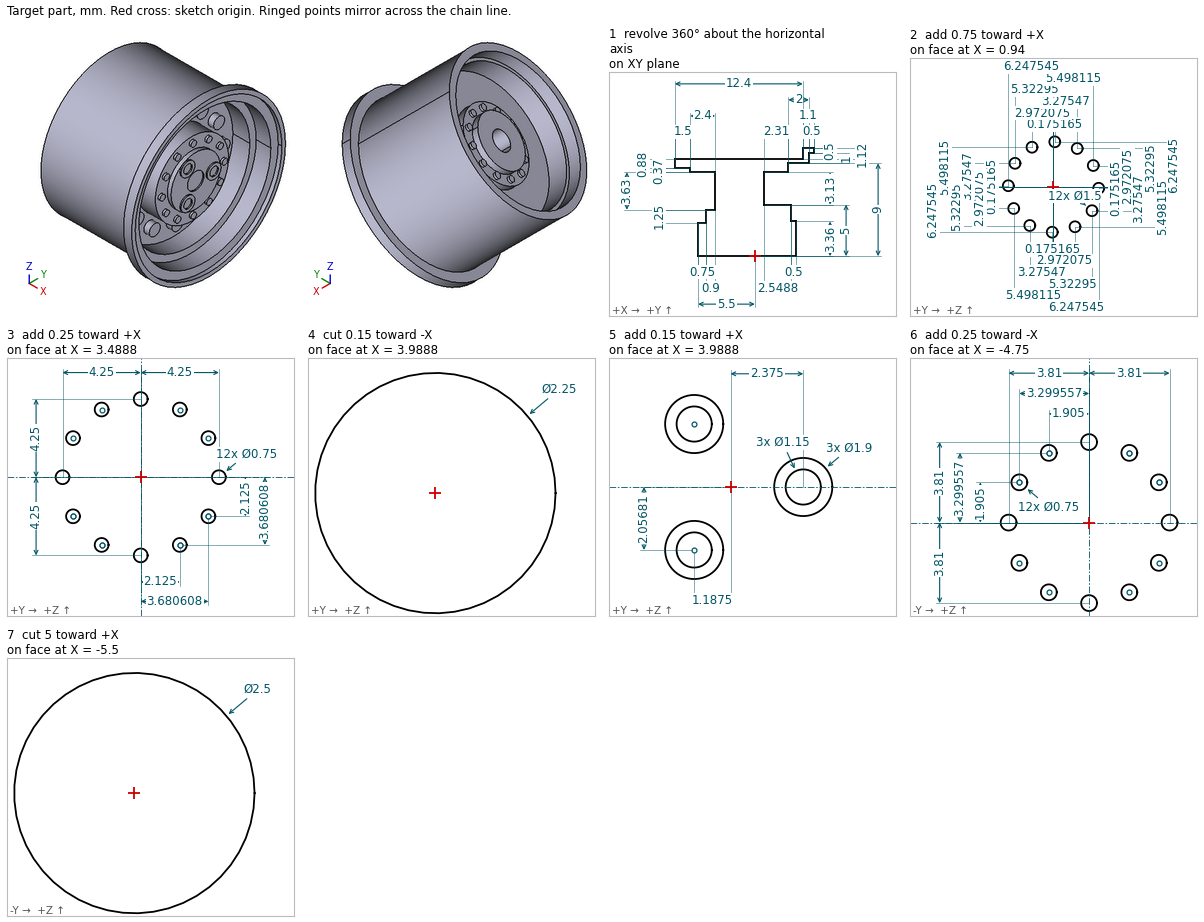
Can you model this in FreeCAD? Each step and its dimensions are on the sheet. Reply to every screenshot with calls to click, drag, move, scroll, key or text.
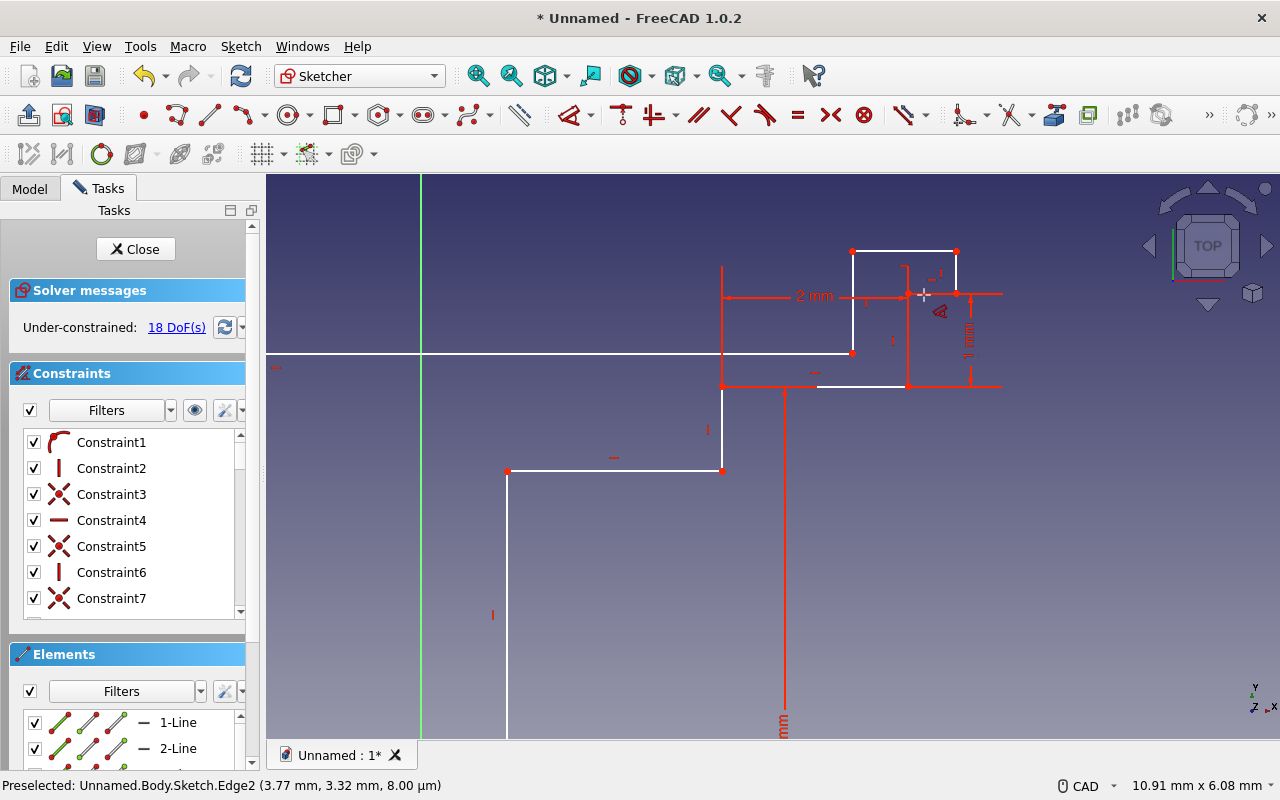
click(922, 294)
click(932, 236)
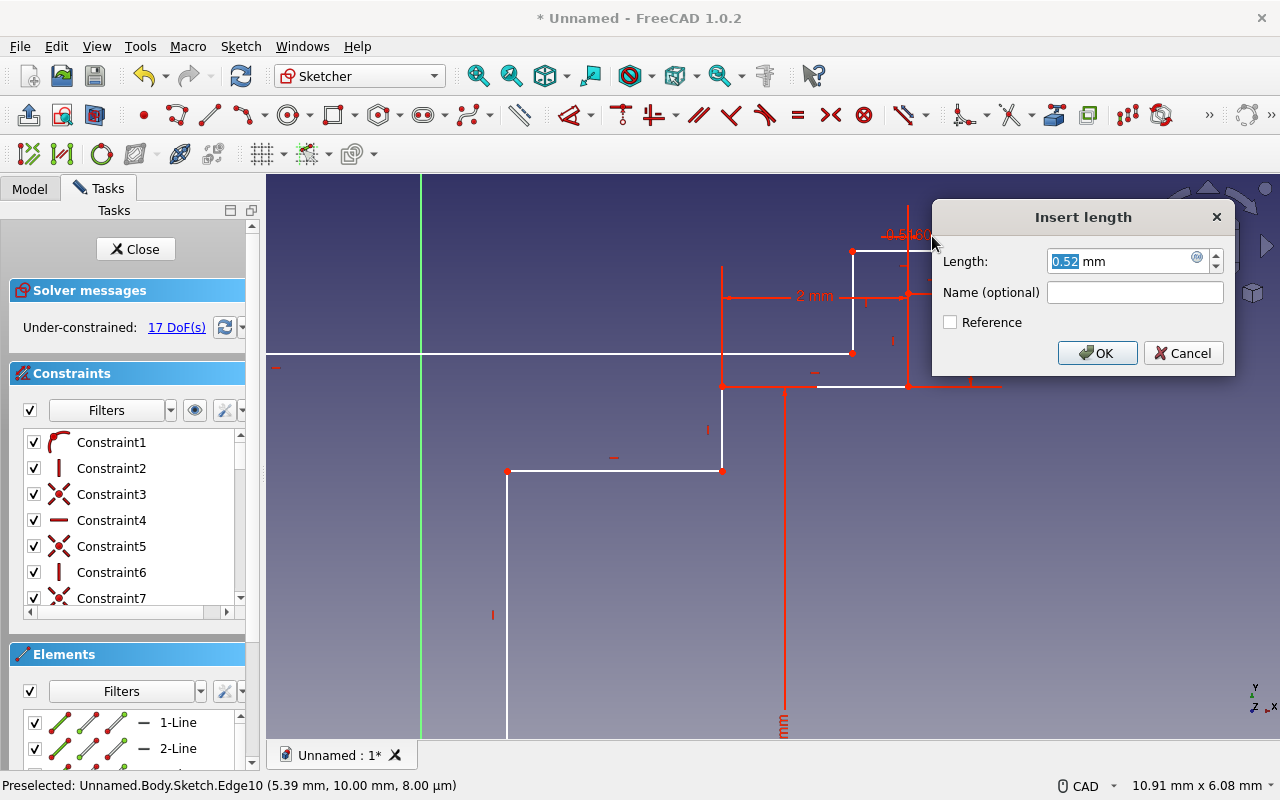
text(0.5)
key(Return)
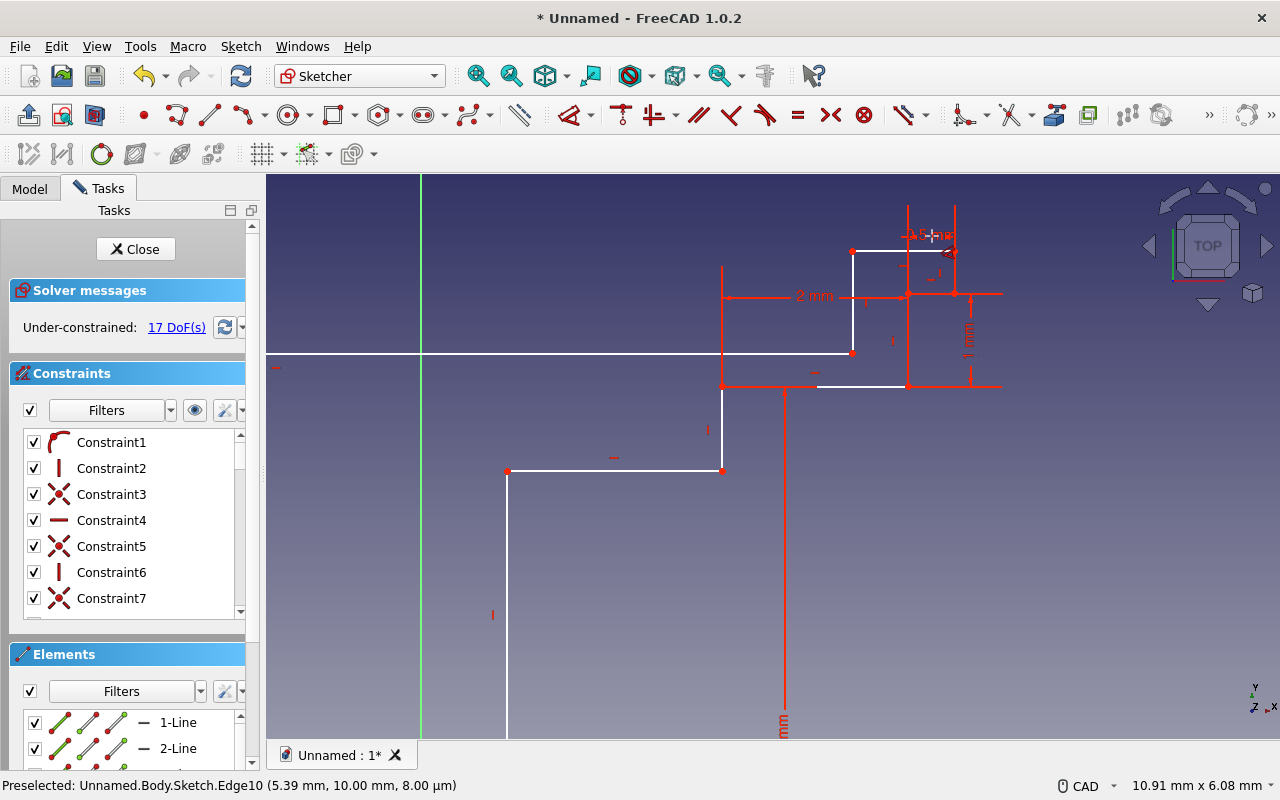
click(955, 281)
click(989, 273)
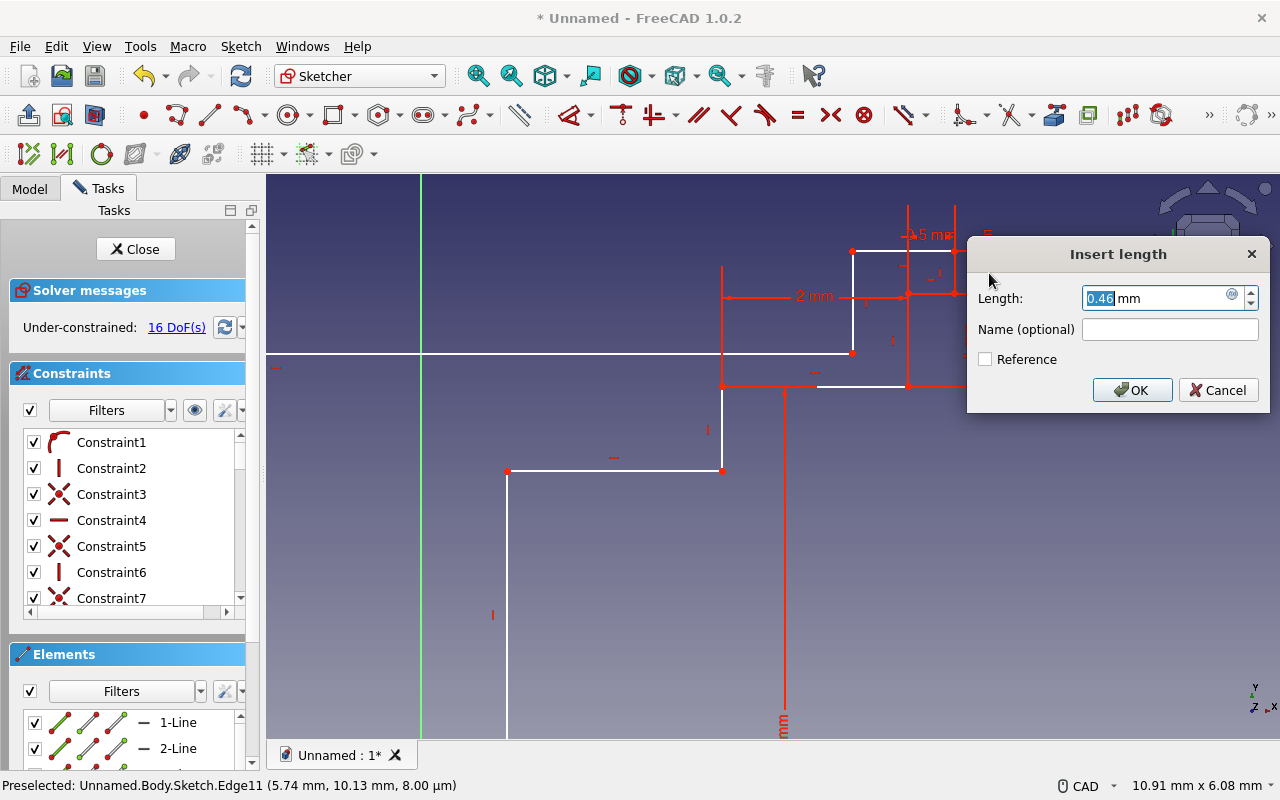
text(0.5)
key(Return)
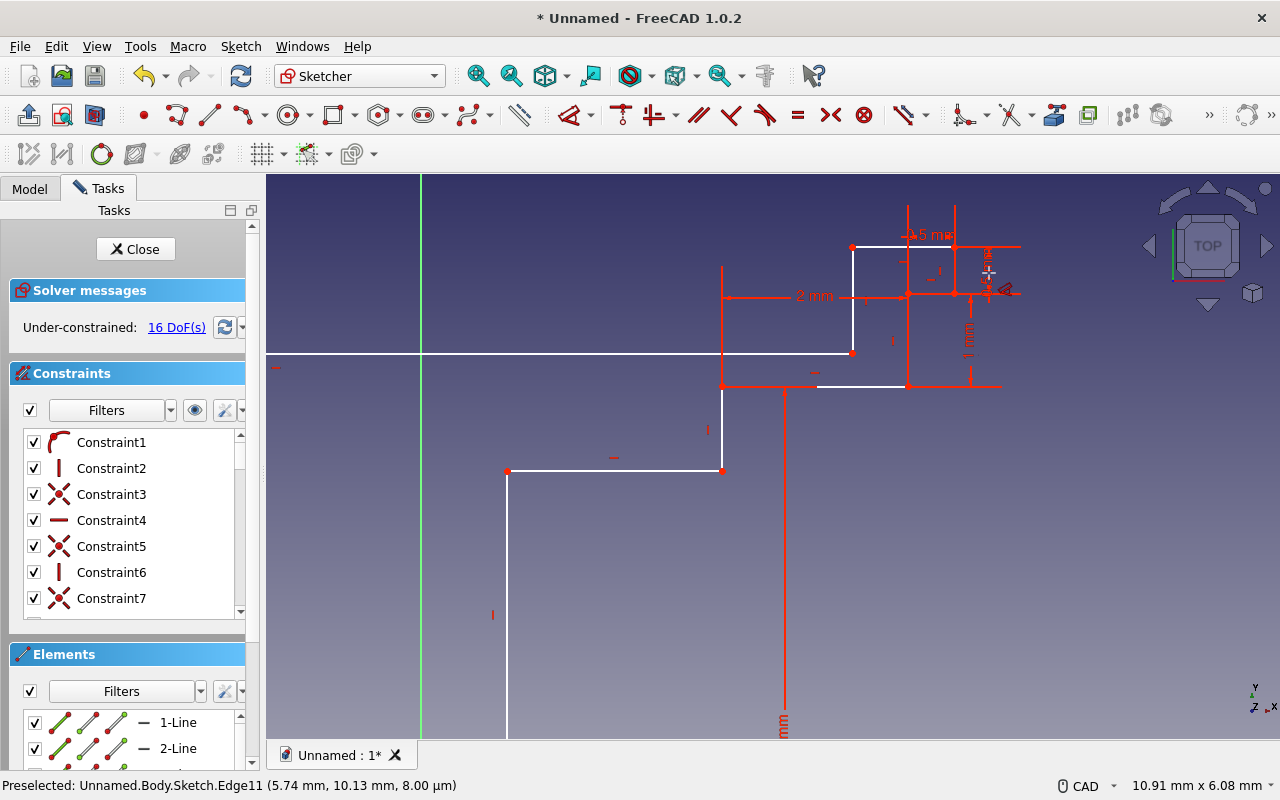
click(924, 247)
click(904, 213)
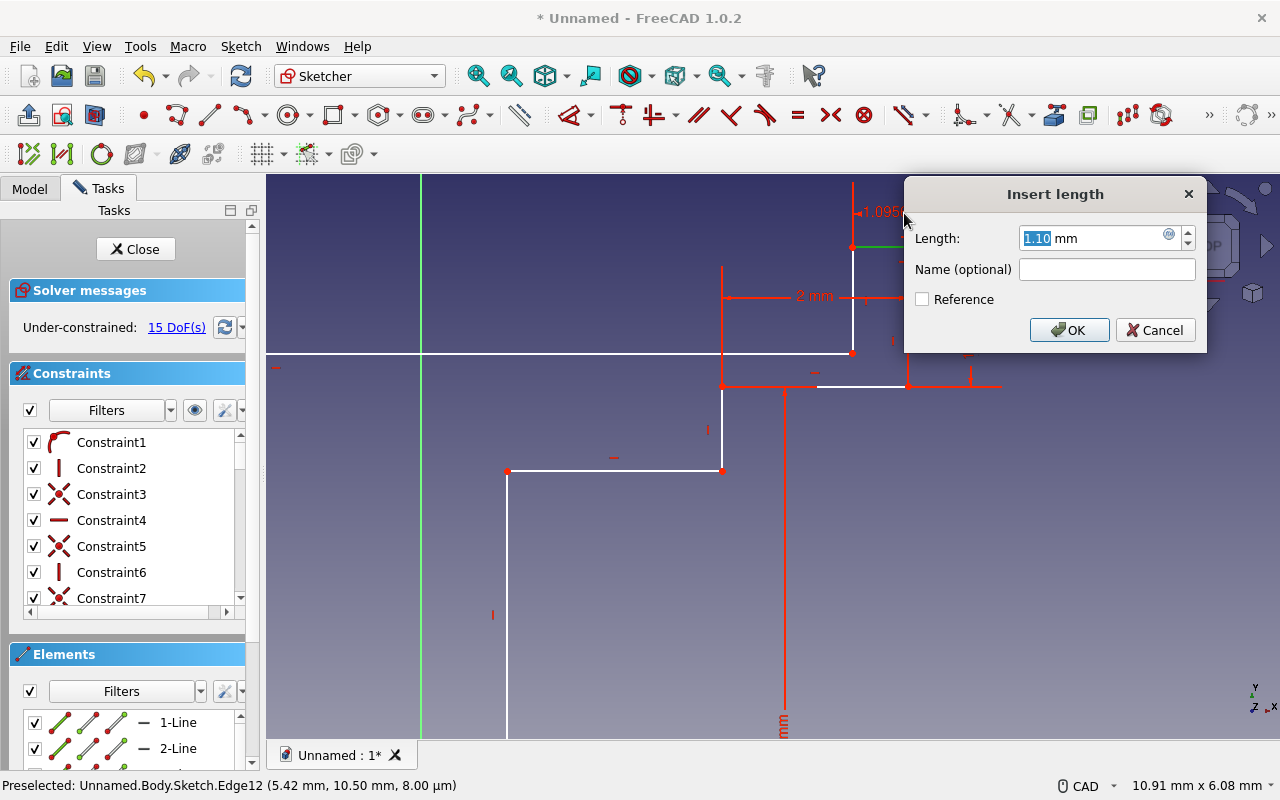
text(1.1)
key(Return)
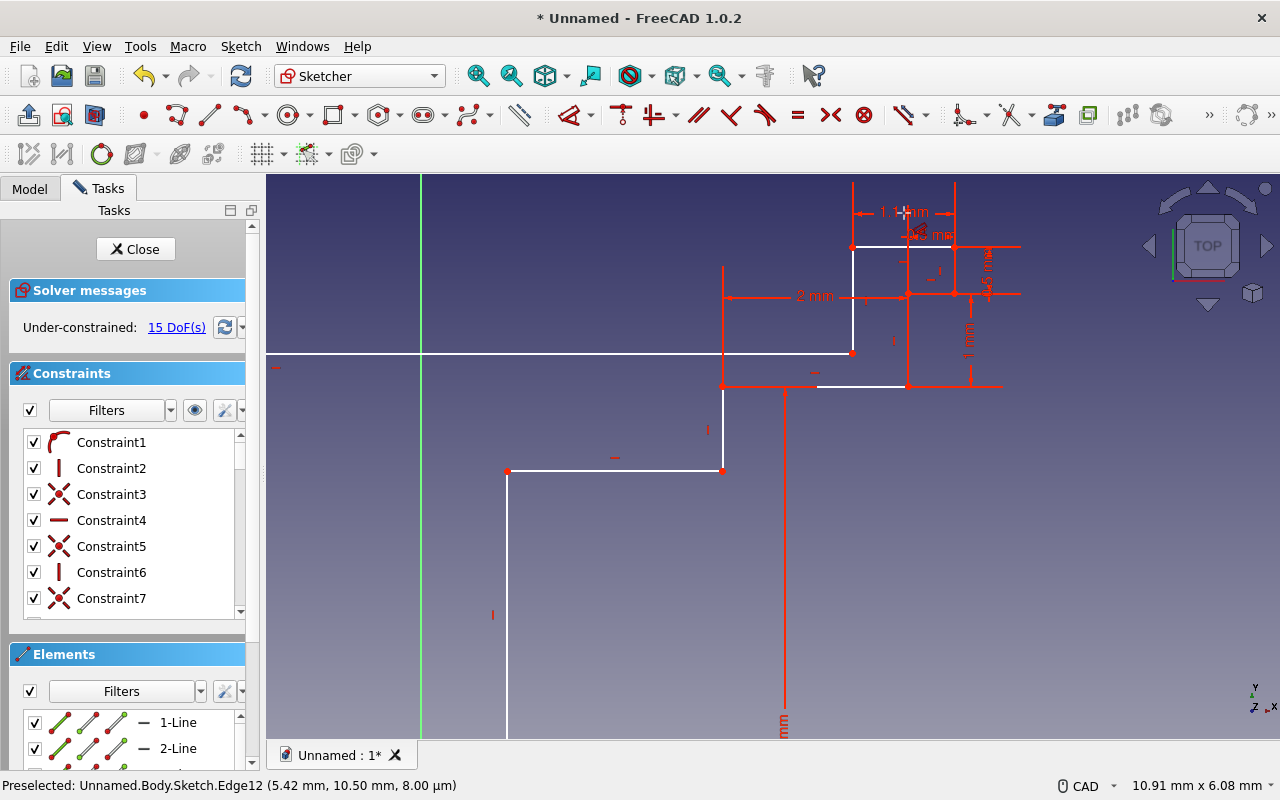
scroll(924, 294, down, 5)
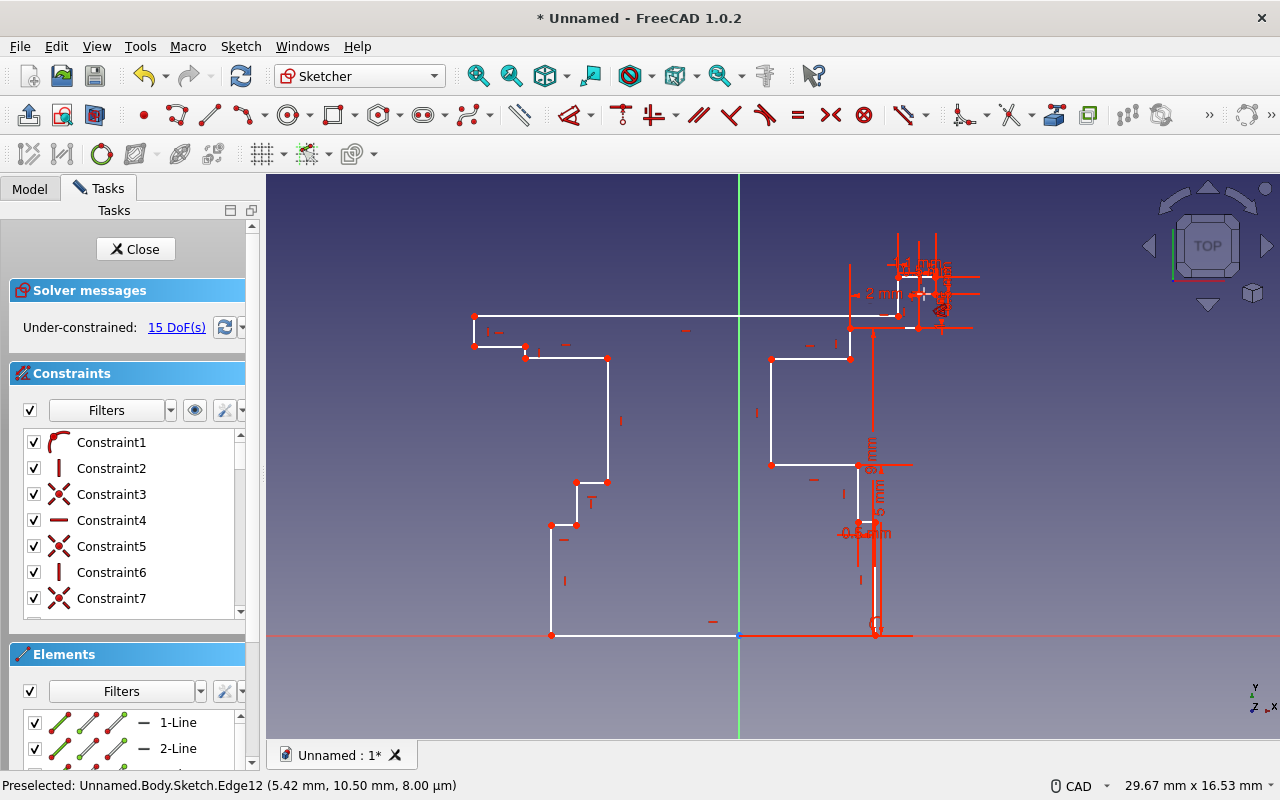
click(490, 347)
click(500, 381)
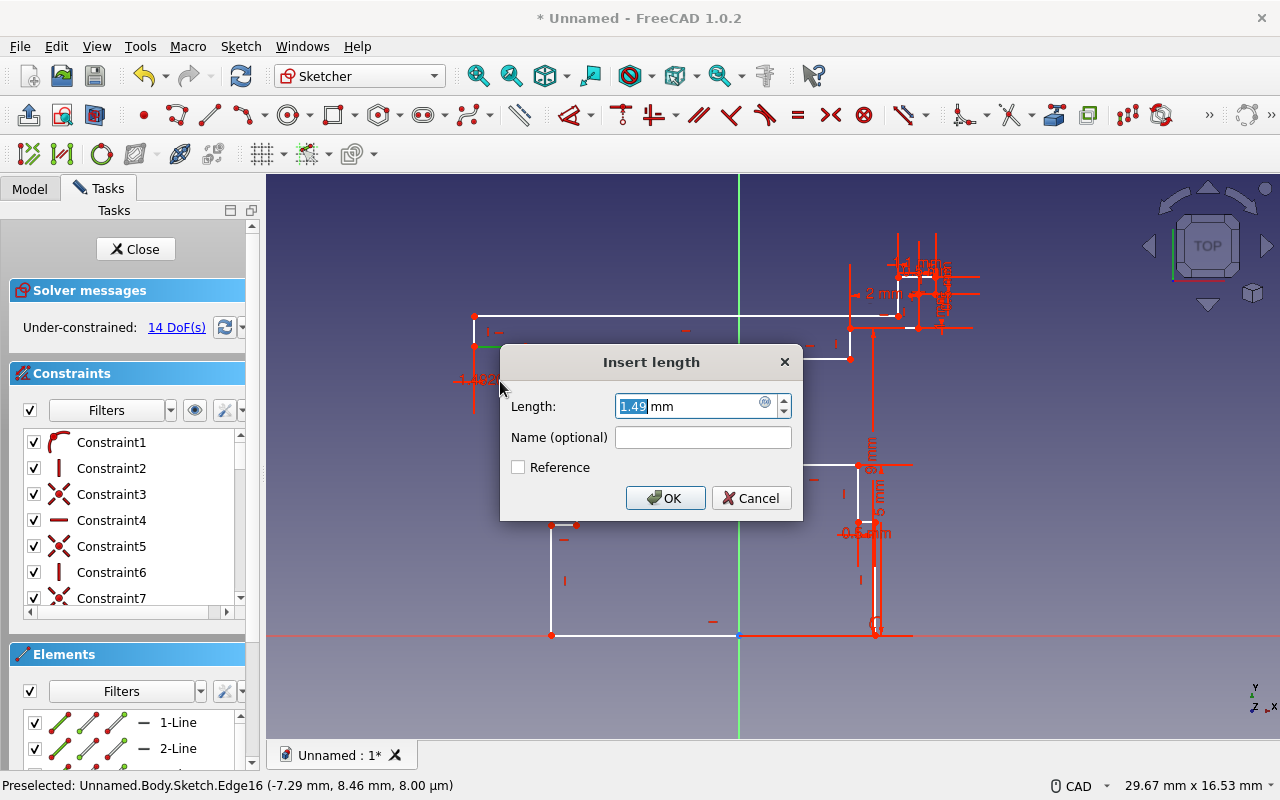
text(1.5)
key(Return)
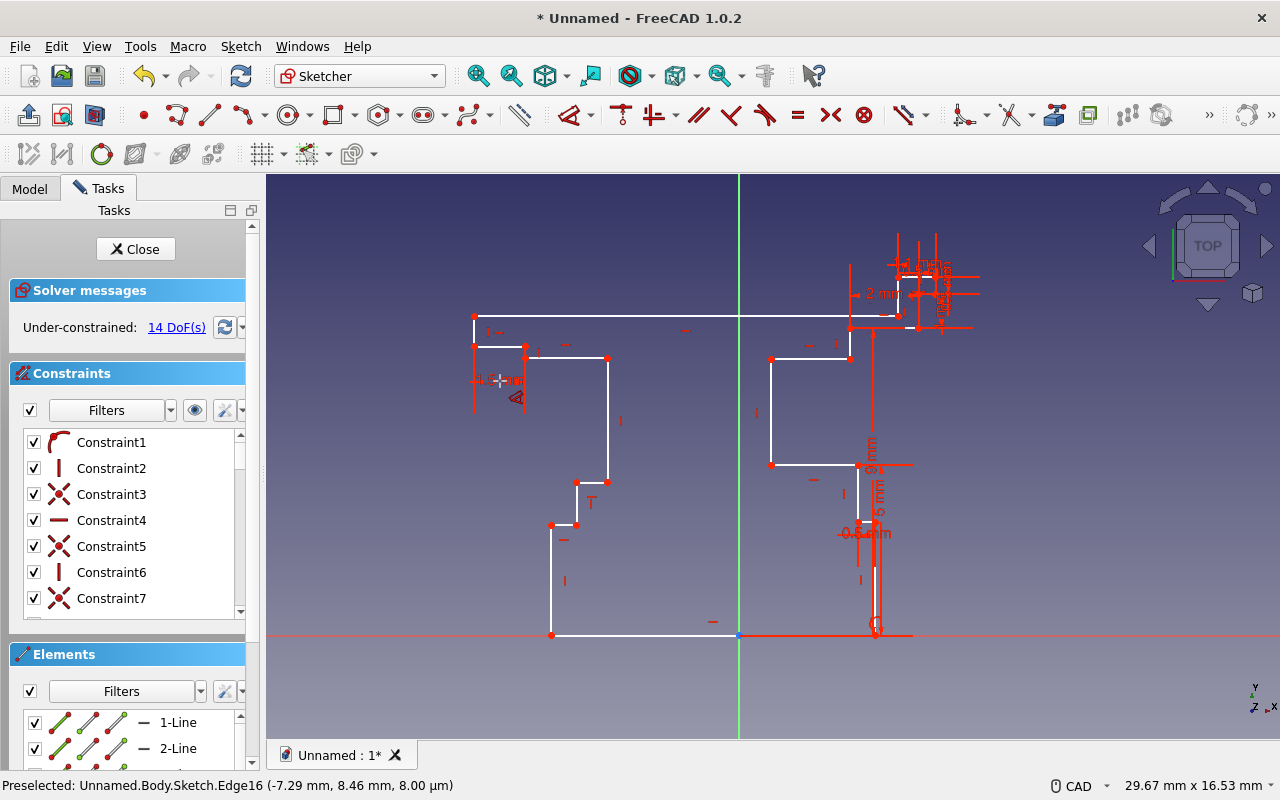
click(550, 358)
click(586, 392)